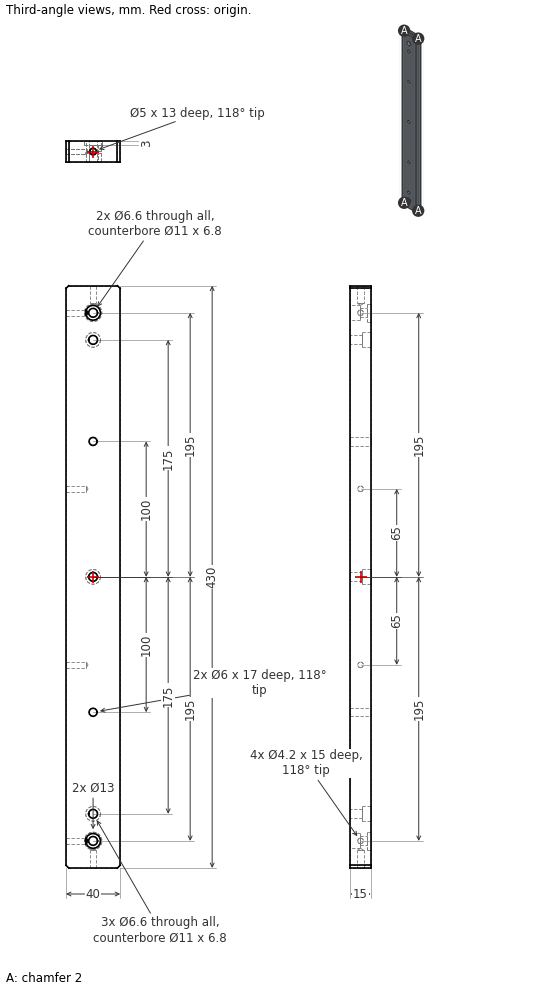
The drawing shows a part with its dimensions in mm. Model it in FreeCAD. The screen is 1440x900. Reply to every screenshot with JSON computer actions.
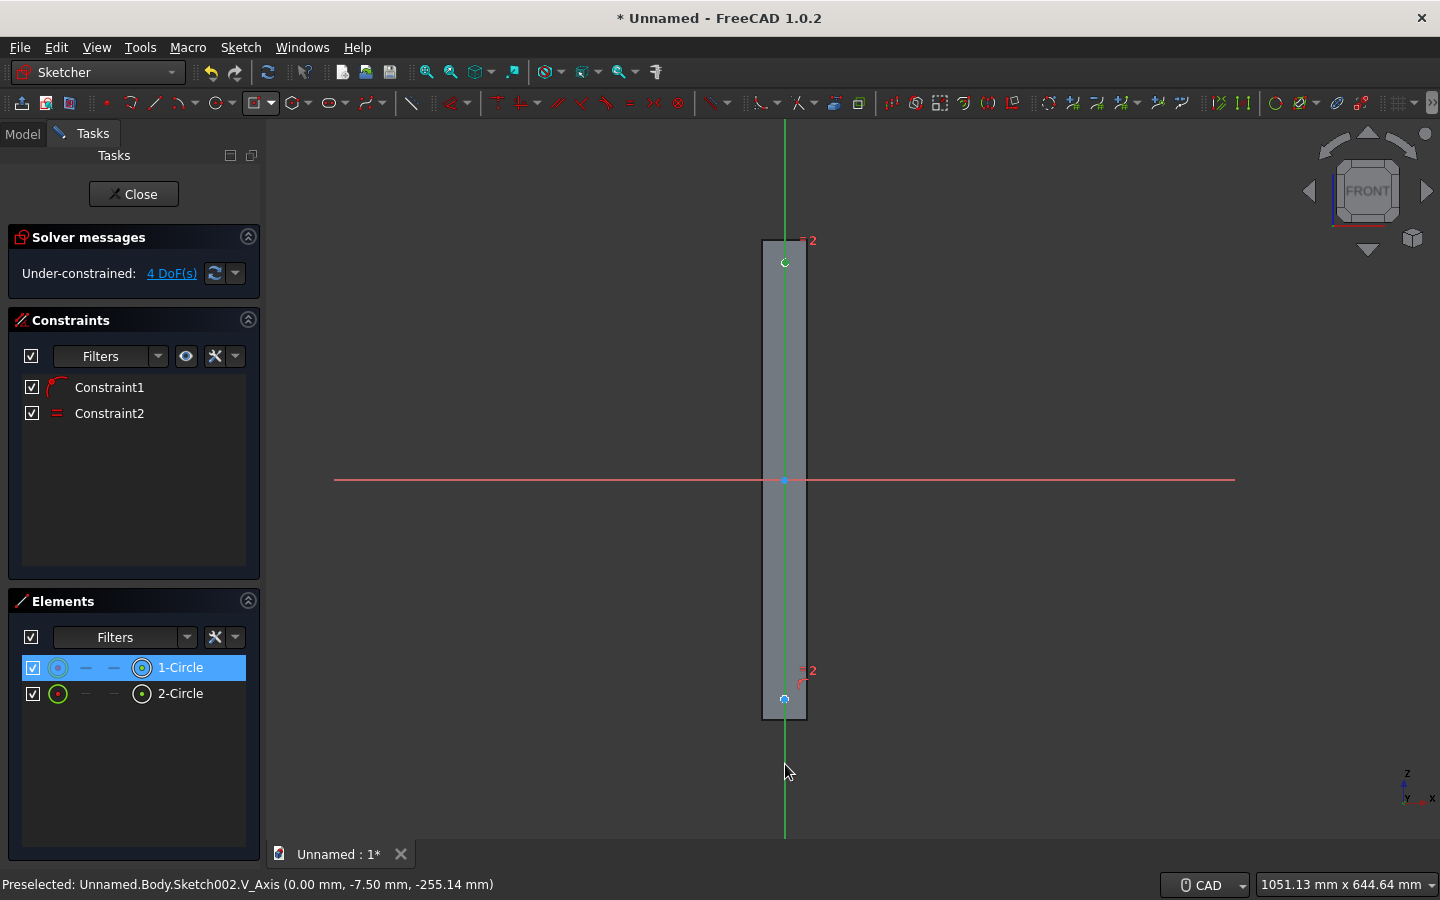
{"action": "key", "text": "c"}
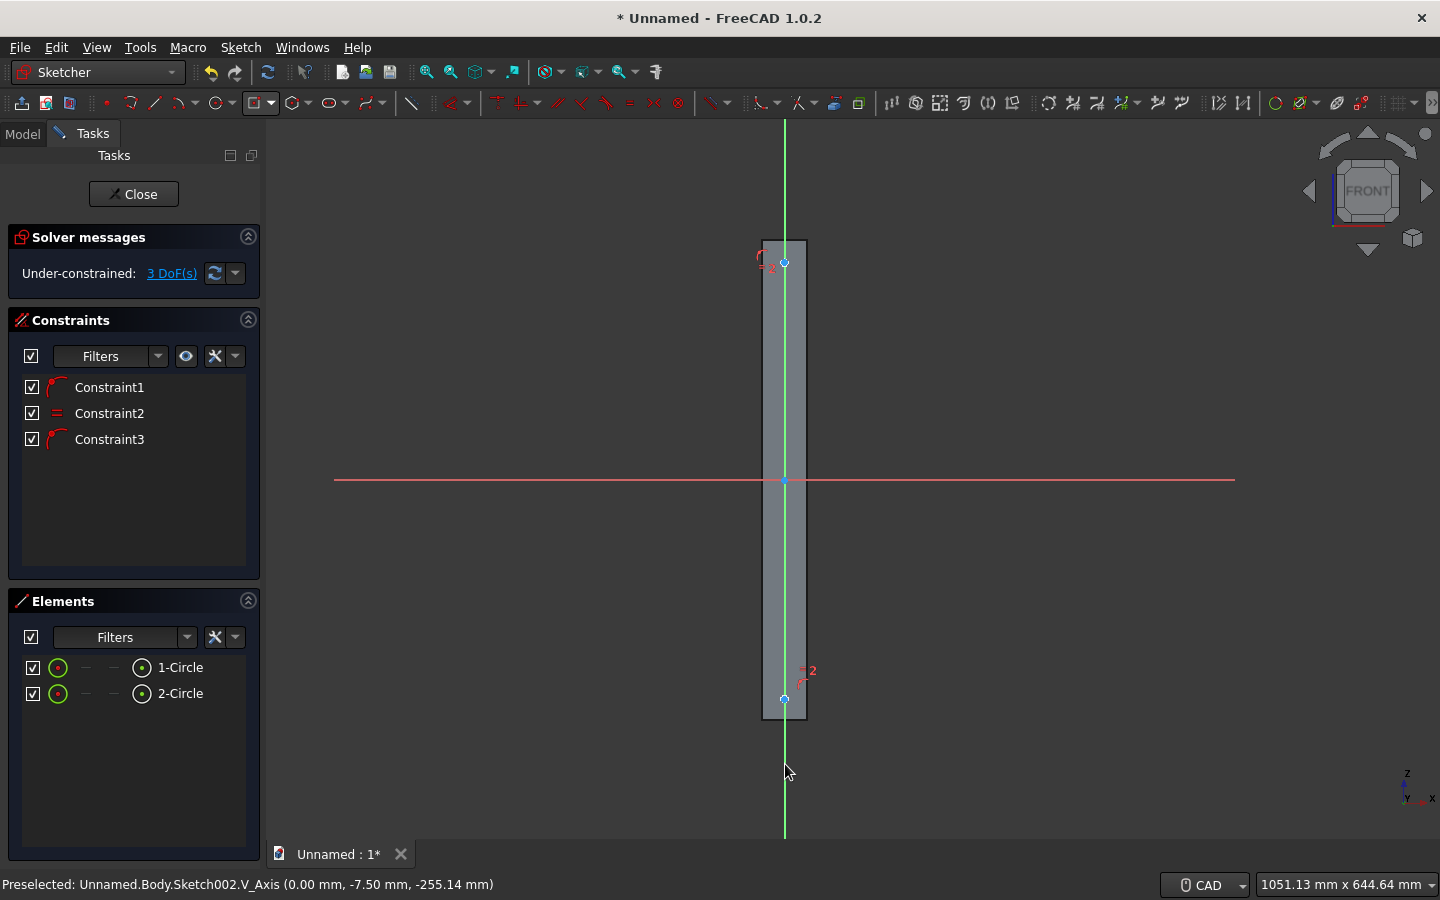
{"action": "key", "text": "d"}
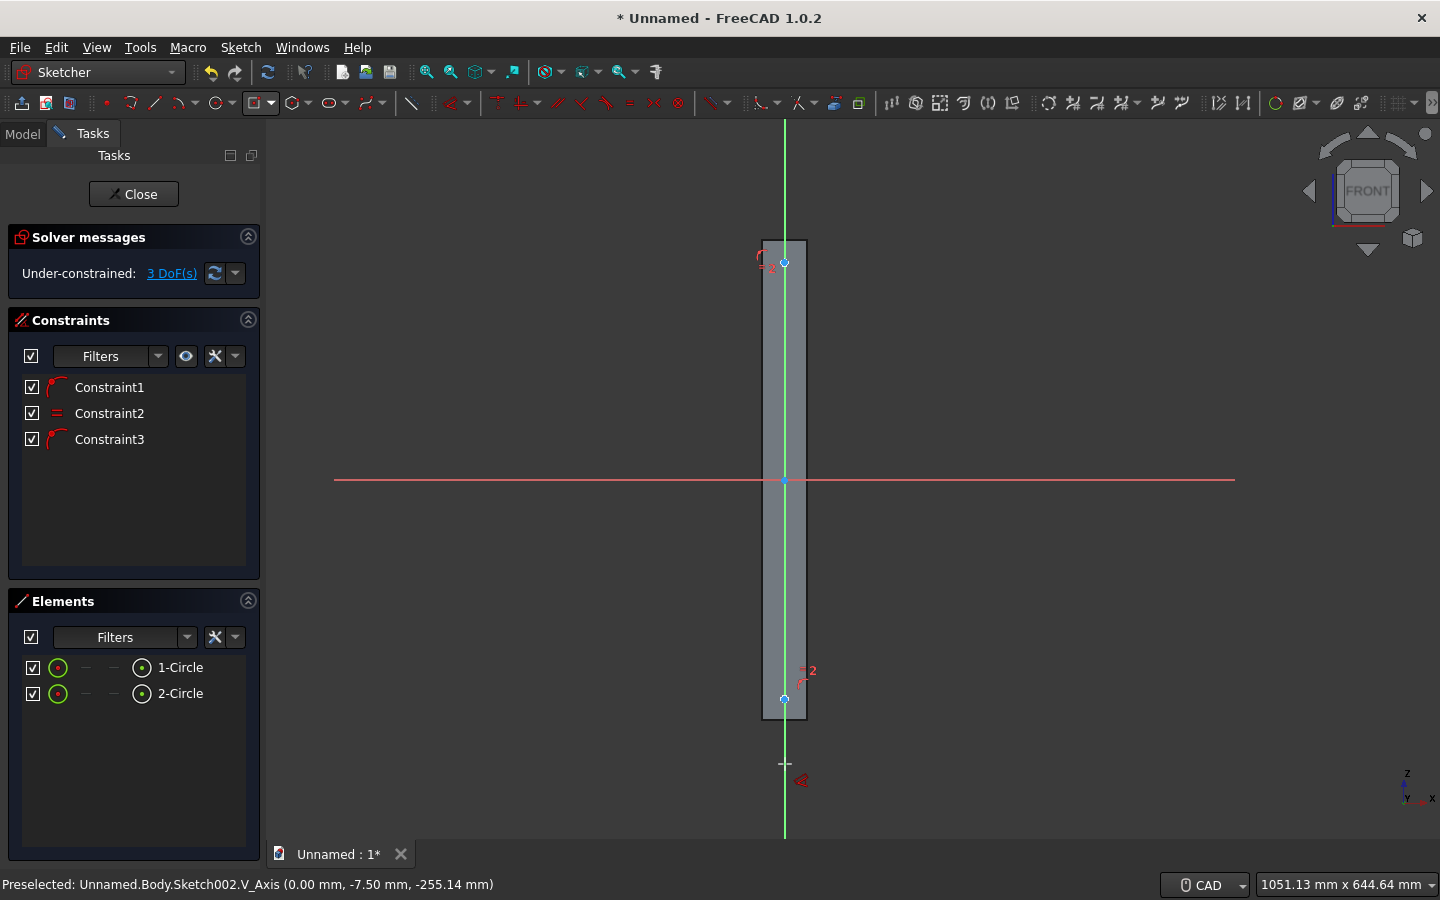
{"action": "scroll", "coordinate": [787, 260], "scroll_direction": "up", "scroll_amount": 9}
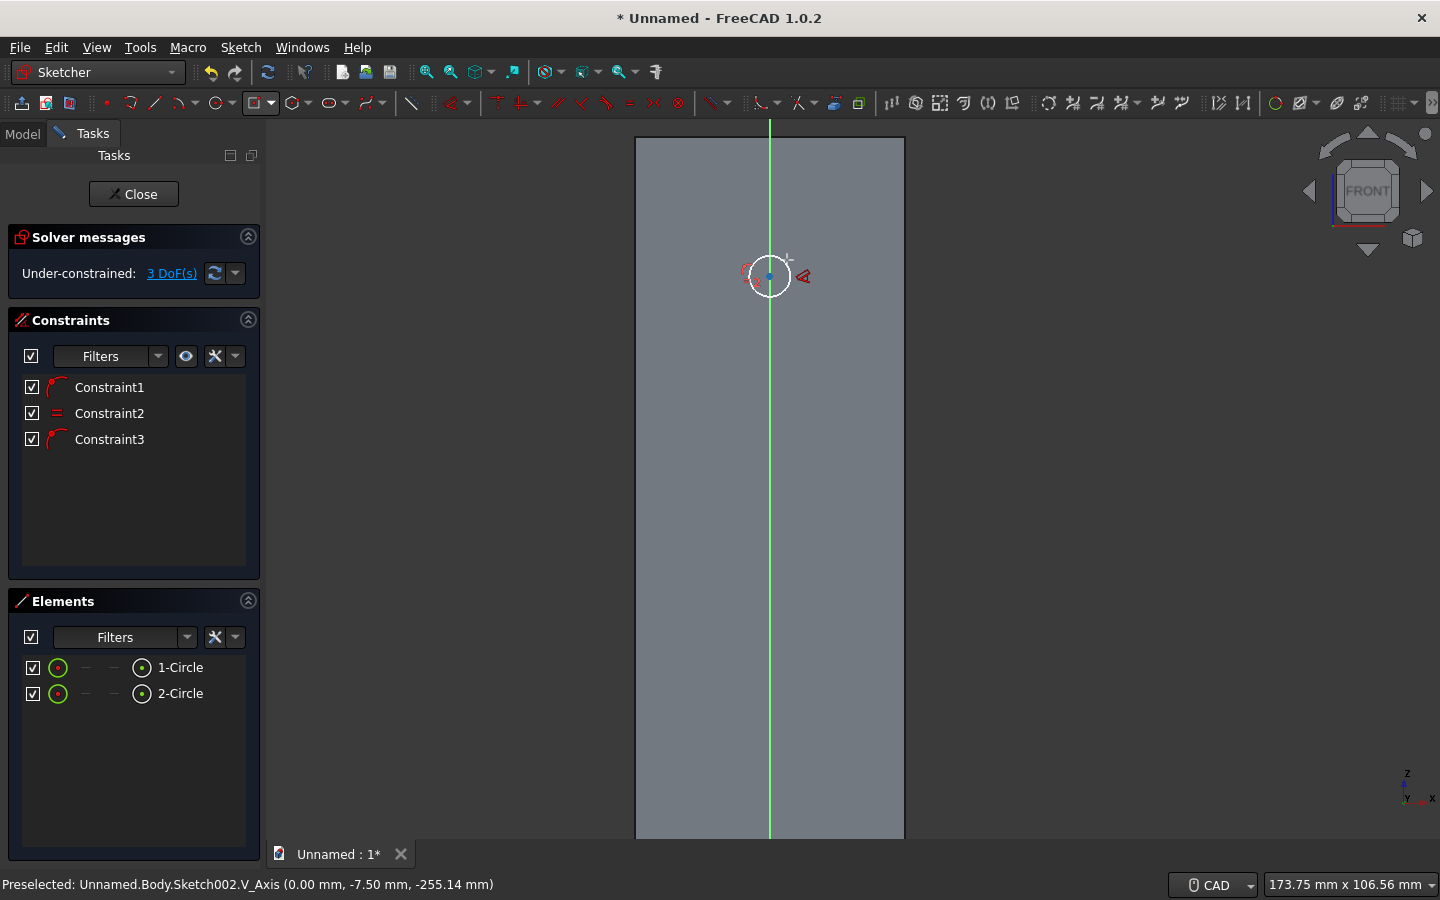
{"action": "left_click", "coordinate": [784, 262]}
{"action": "left_click", "coordinate": [806, 239]}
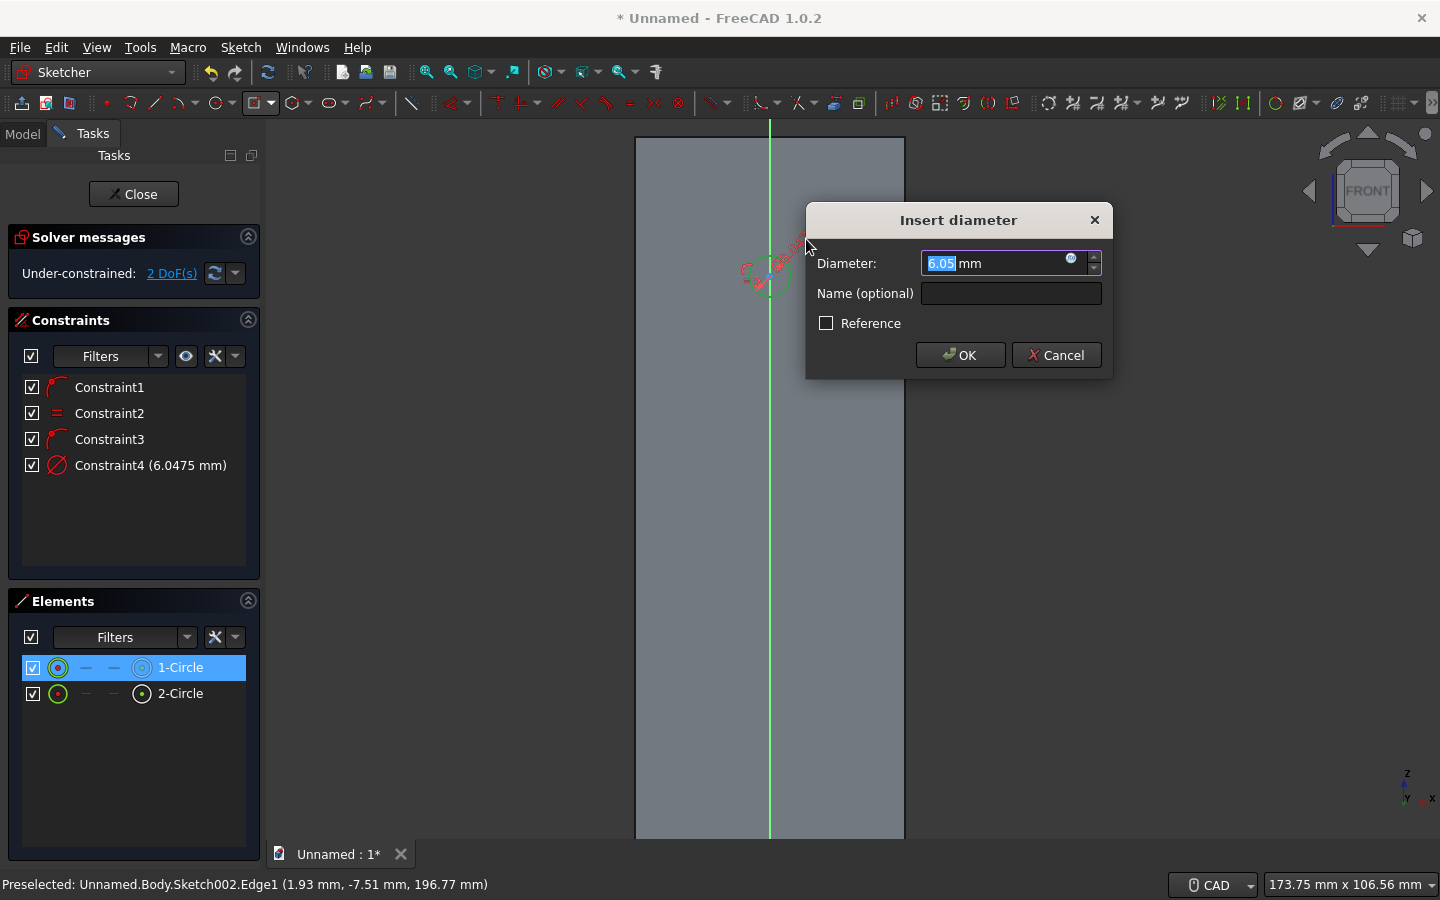
{"action": "type", "text": "6.6"}
{"action": "key", "text": "Return"}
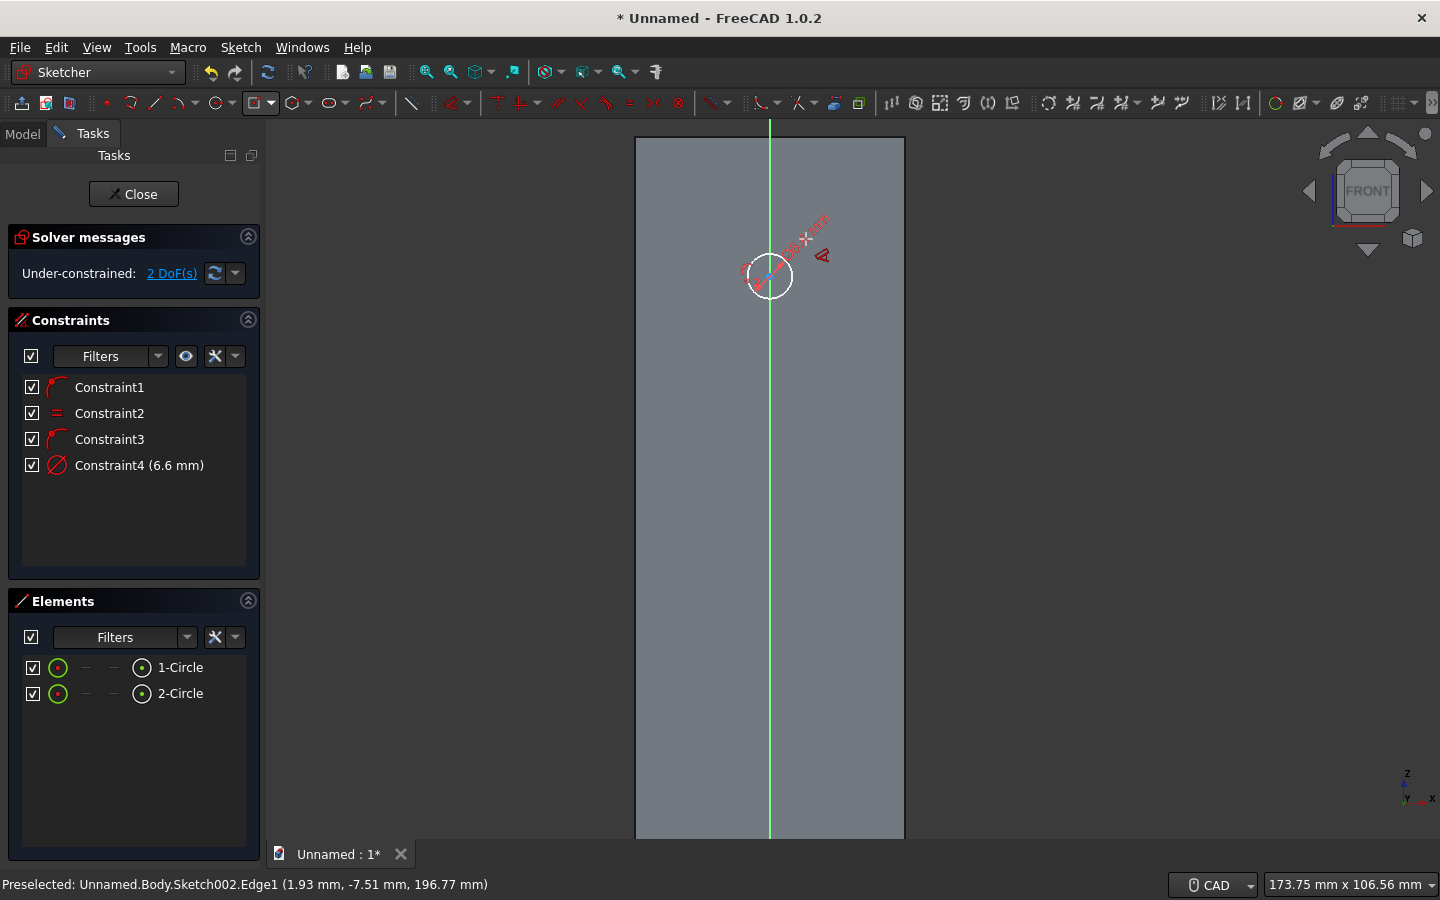
{"action": "scroll", "coordinate": [787, 259], "scroll_direction": "down", "scroll_amount": 9}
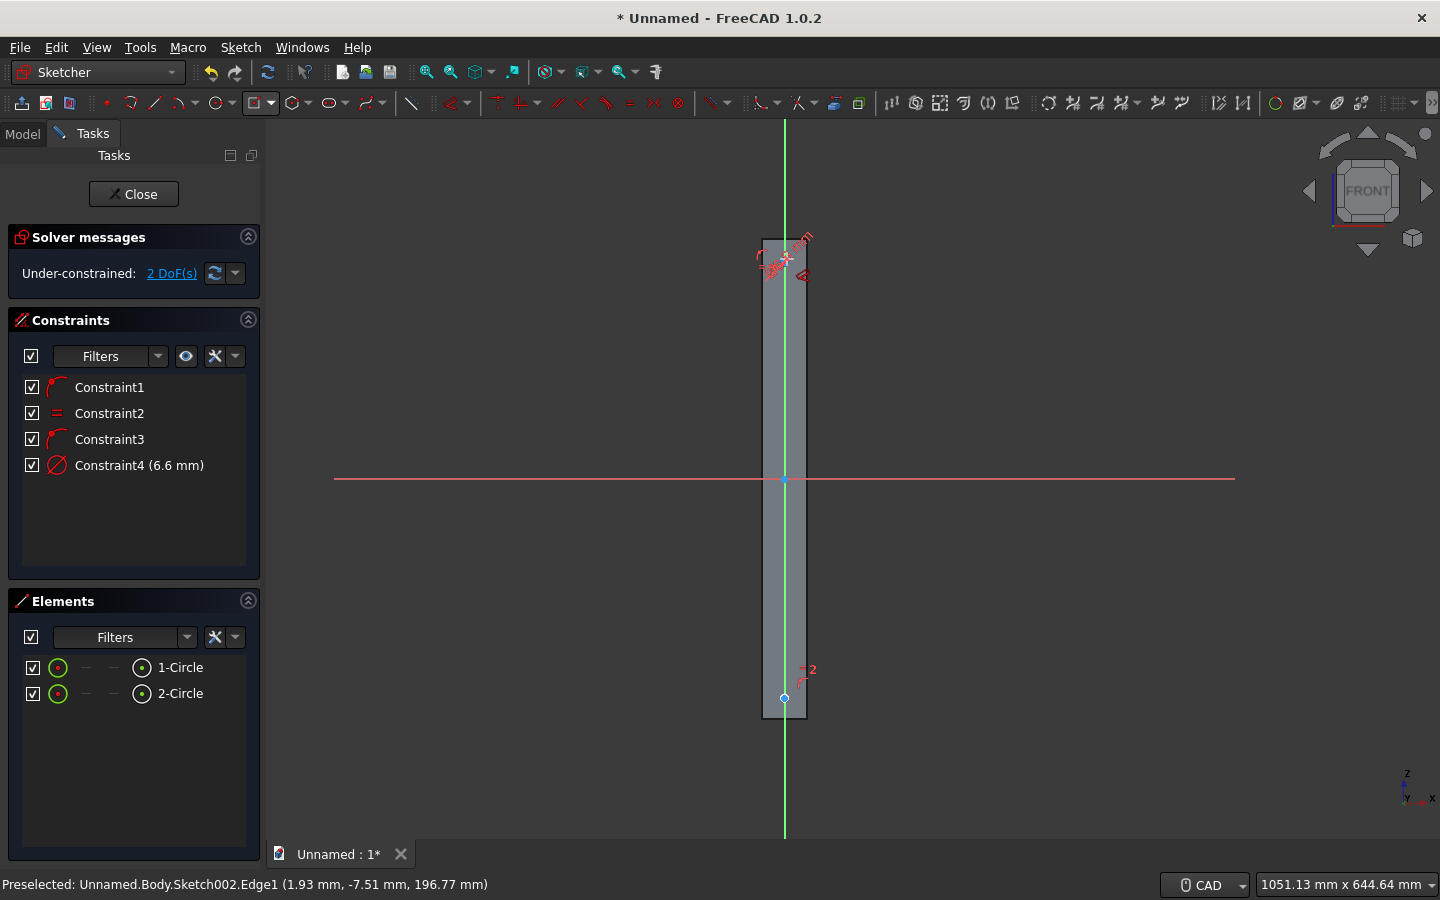
{"action": "left_click", "coordinate": [785, 262]}
{"action": "left_click", "coordinate": [819, 371]}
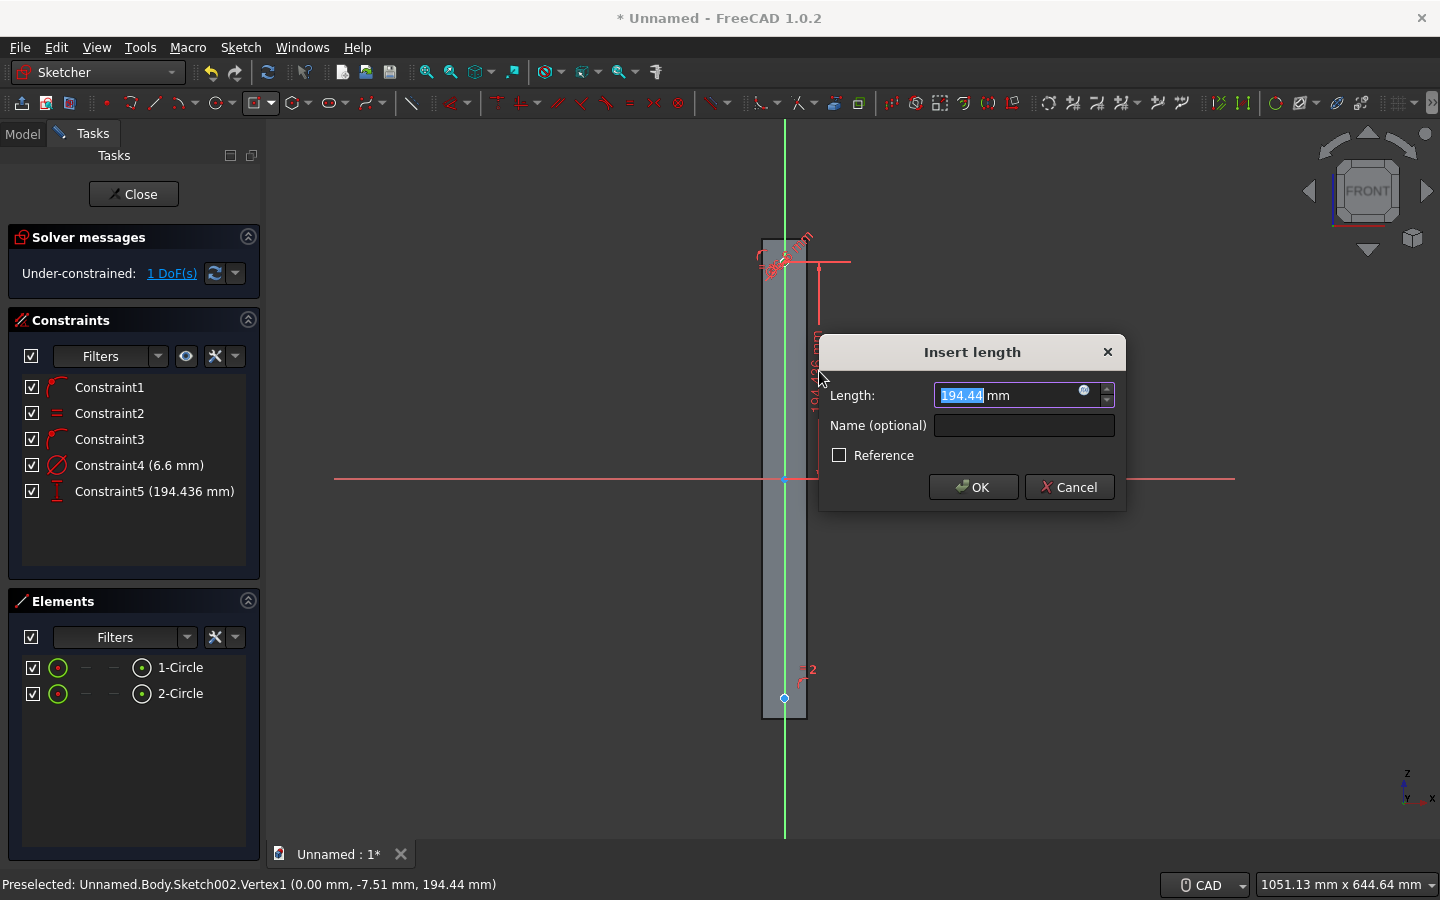
{"action": "type", "text": "195"}
{"action": "key", "text": "Return"}